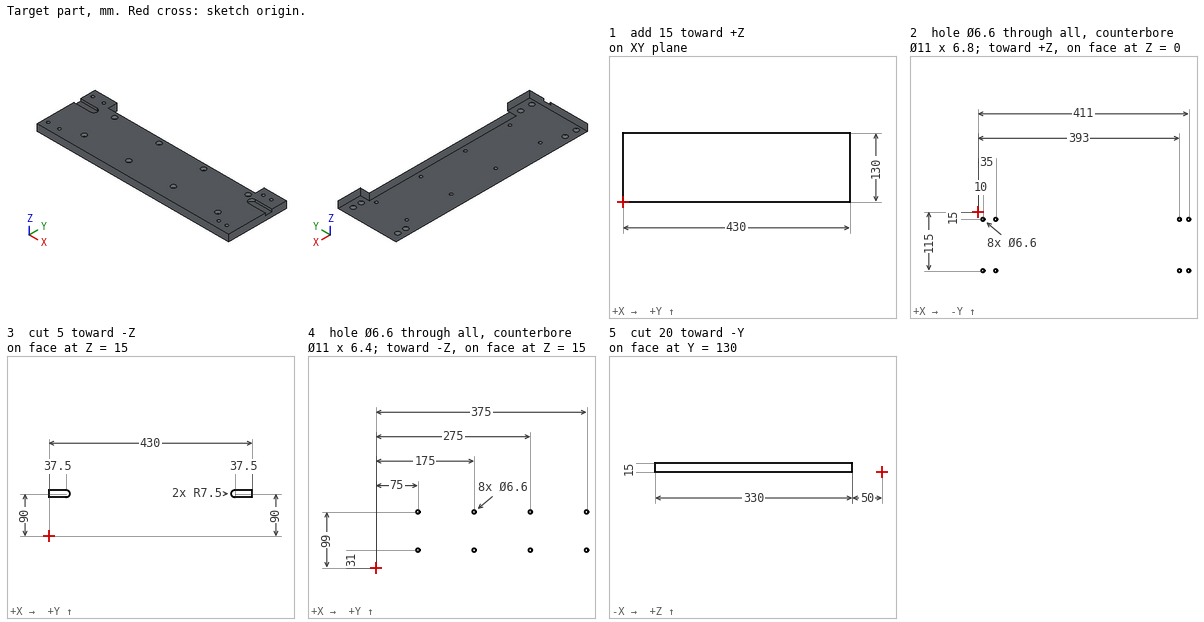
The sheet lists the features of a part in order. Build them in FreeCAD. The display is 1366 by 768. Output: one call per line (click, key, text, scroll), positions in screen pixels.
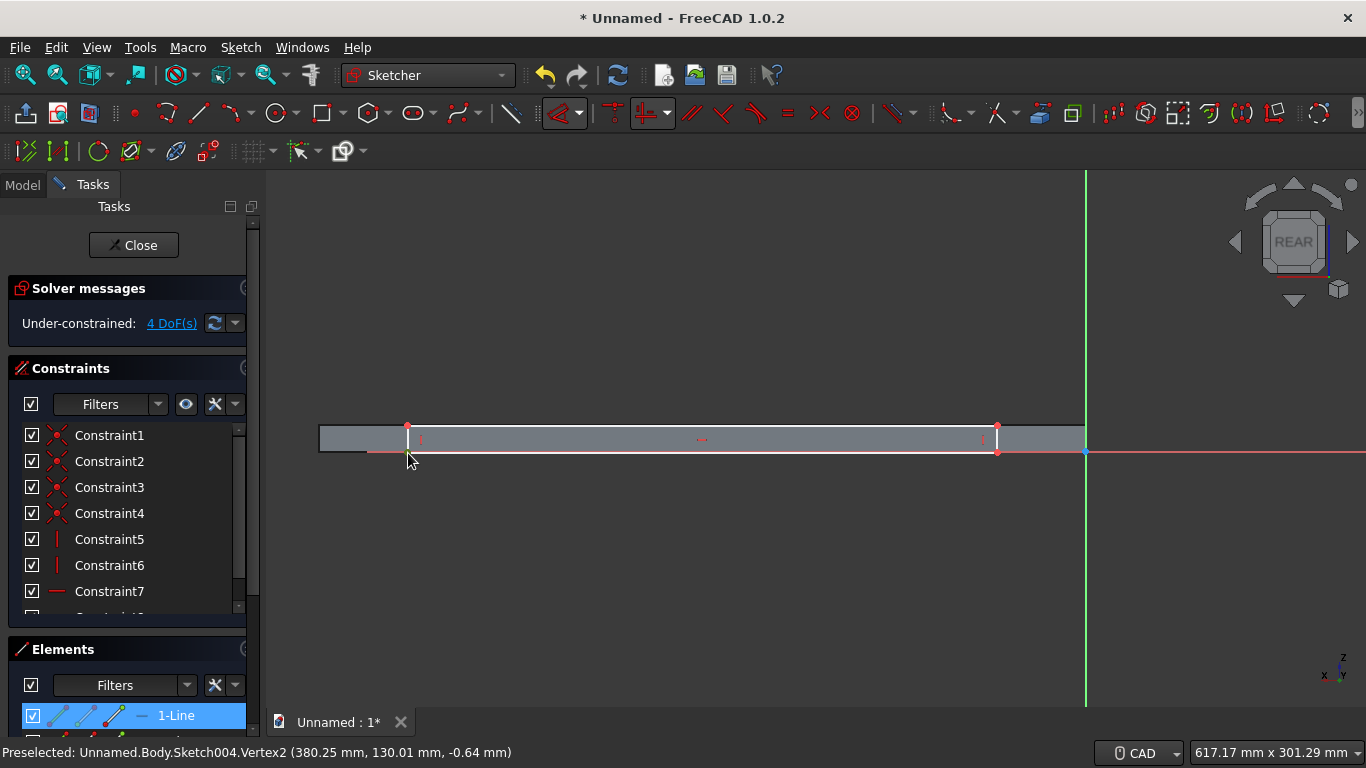
click(1136, 452)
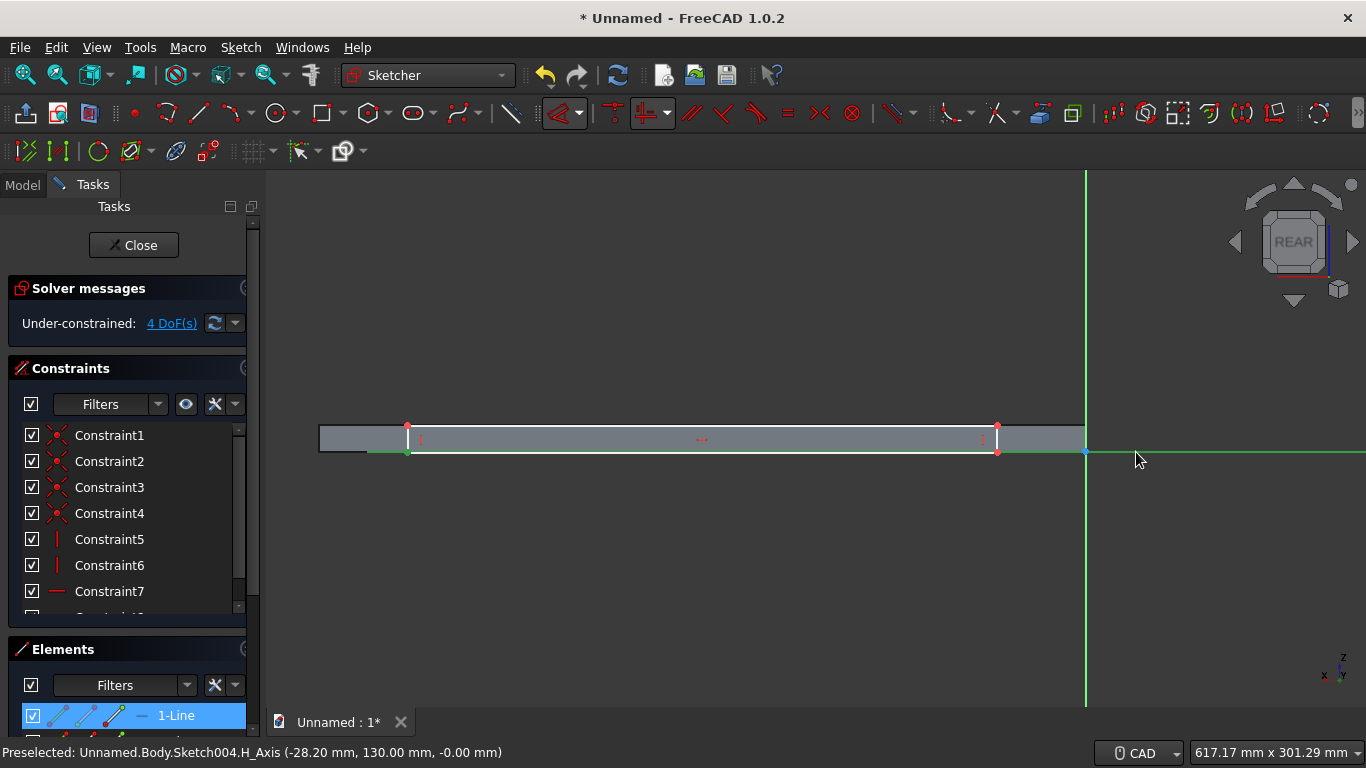
click(614, 114)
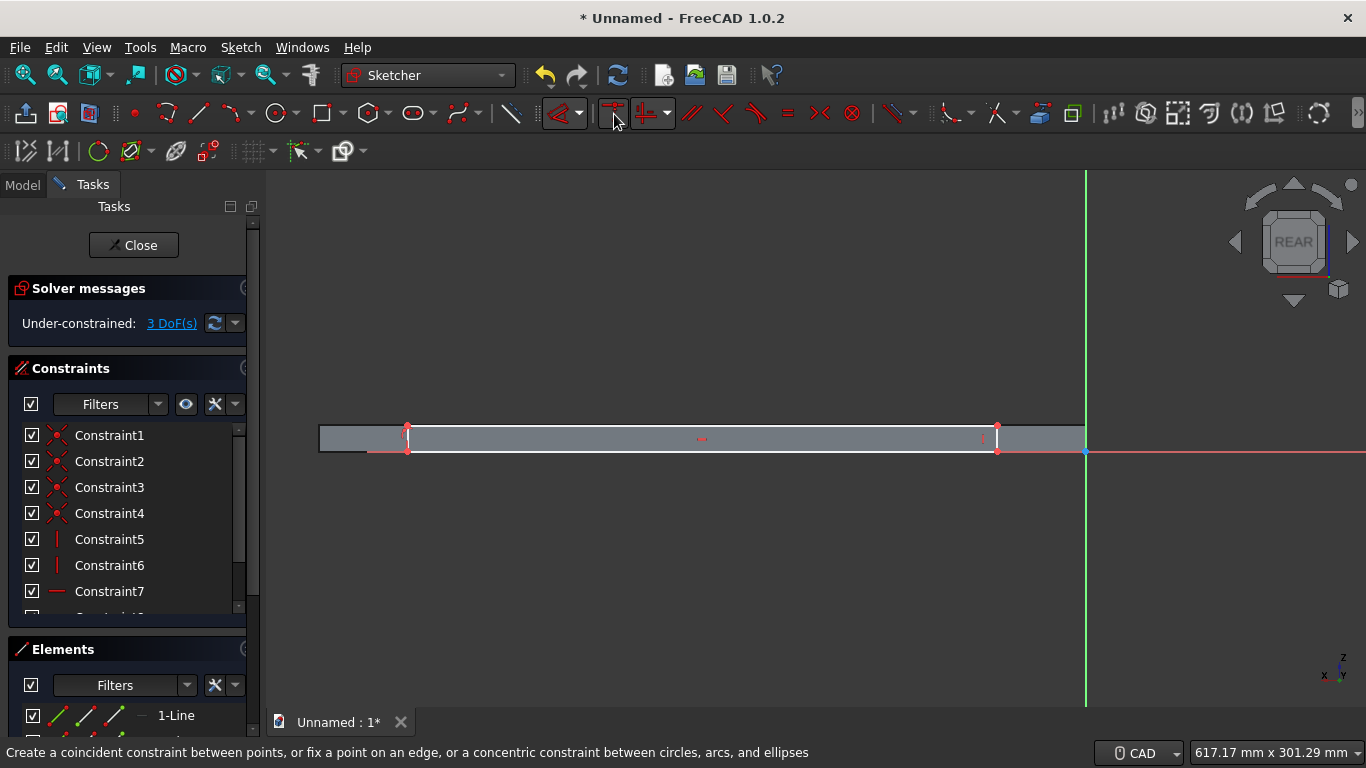
scroll(408, 436, up, 2)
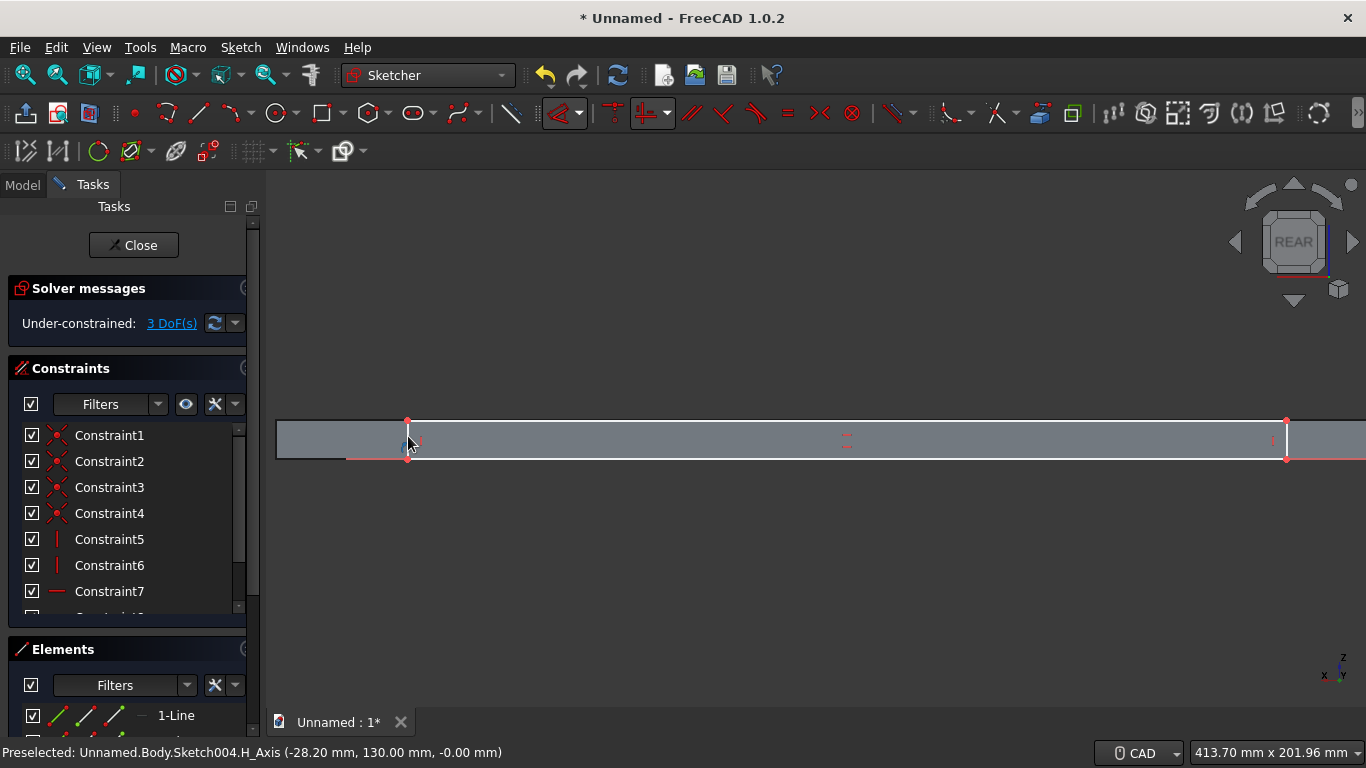
click(408, 436)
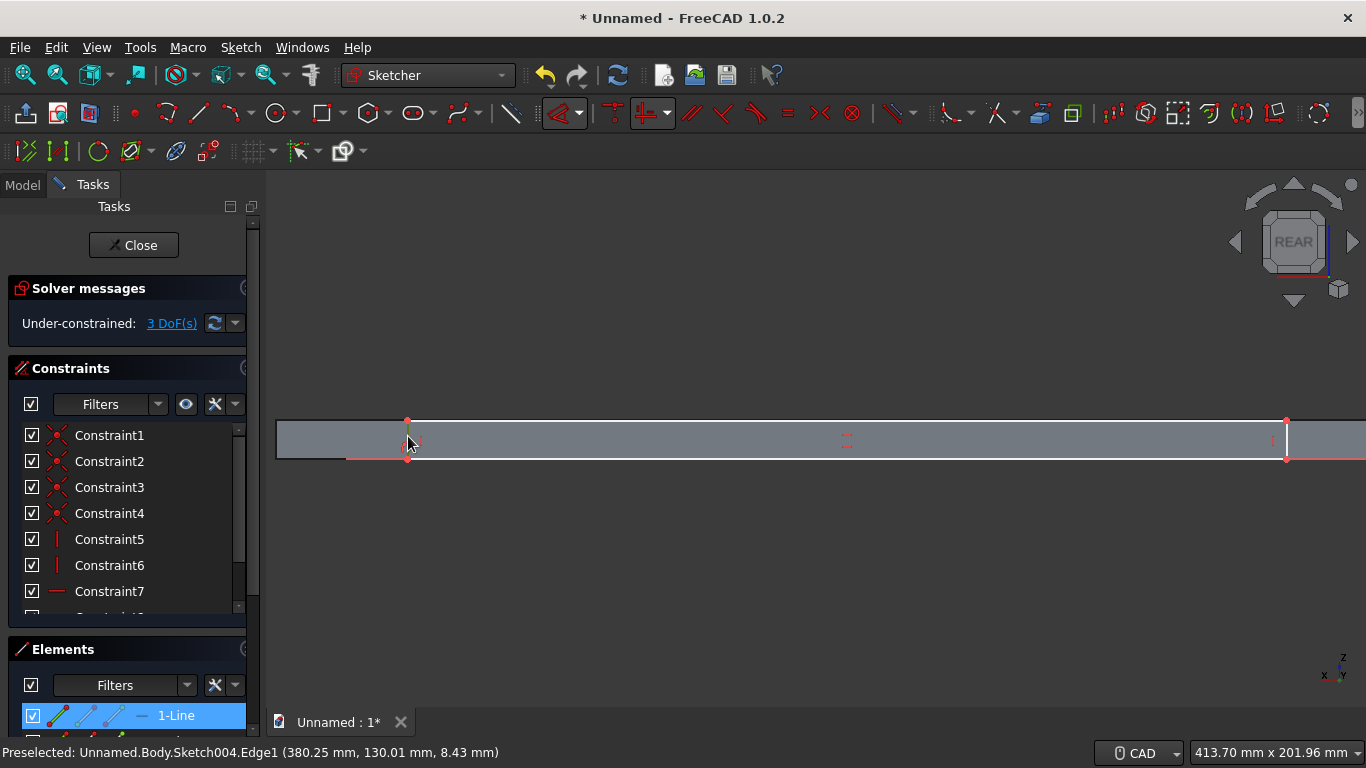
key(i)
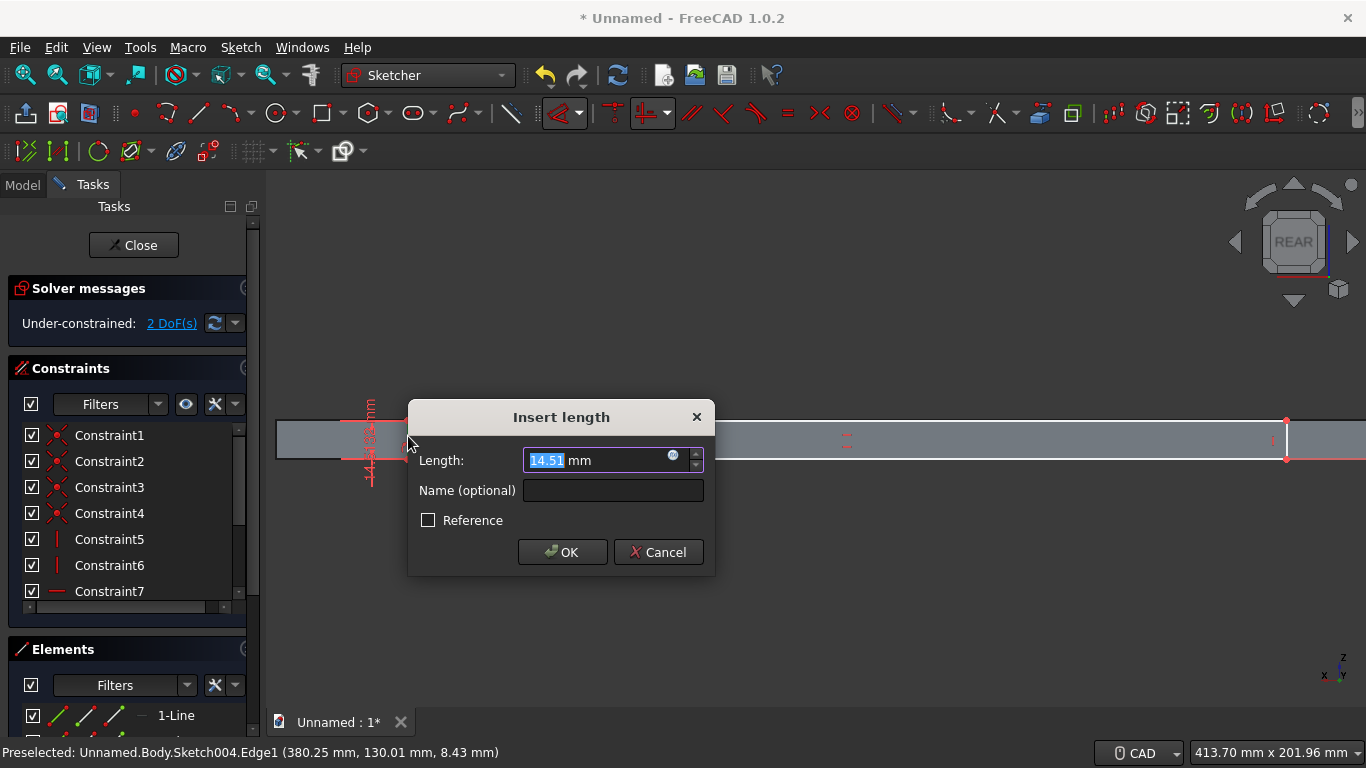
text(15)
key(Return)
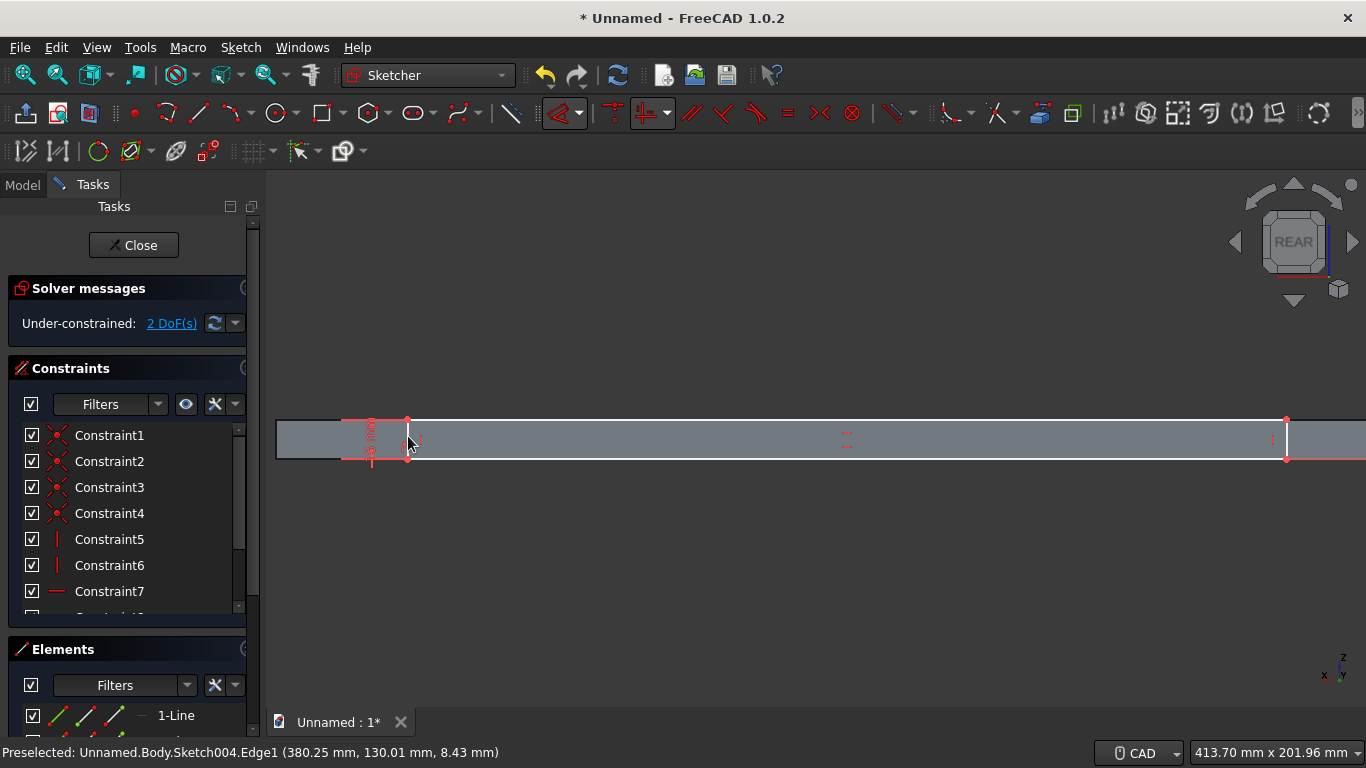
click(672, 459)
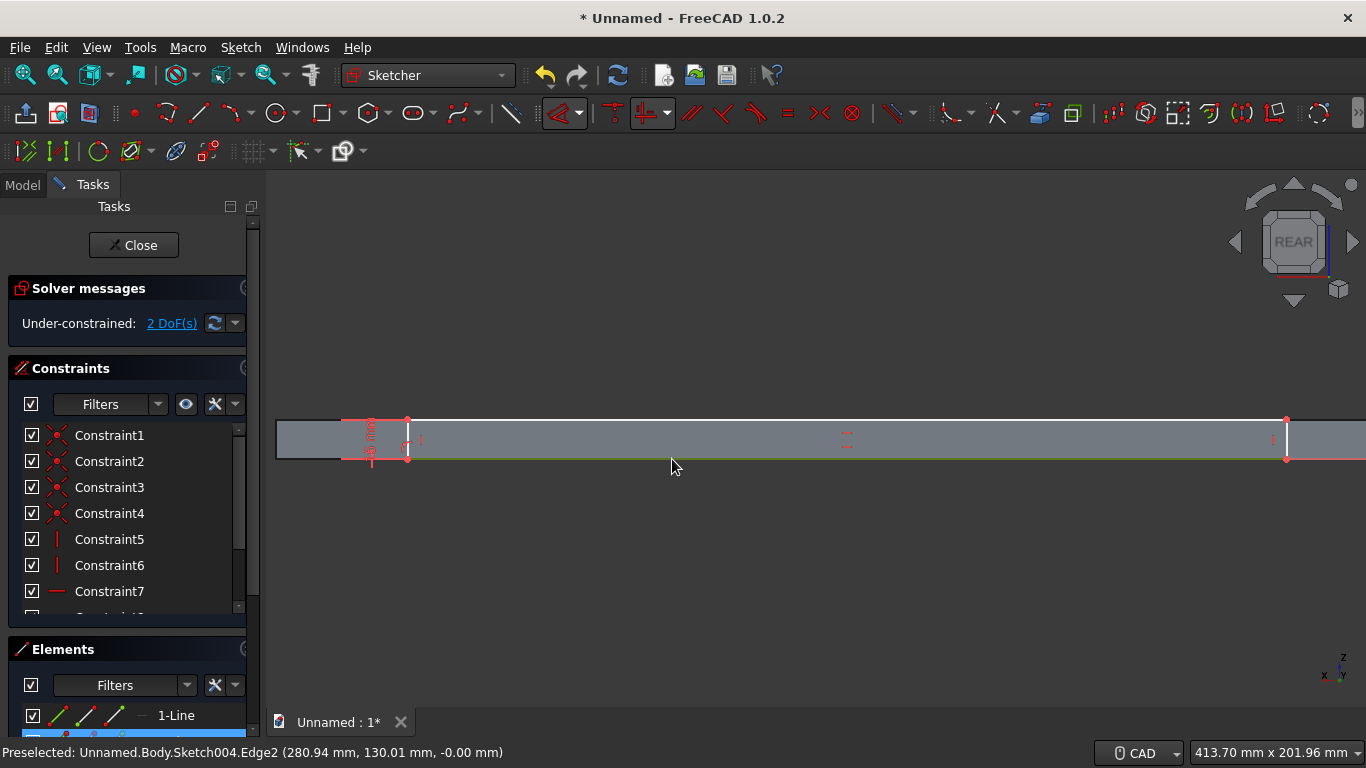
click(582, 114)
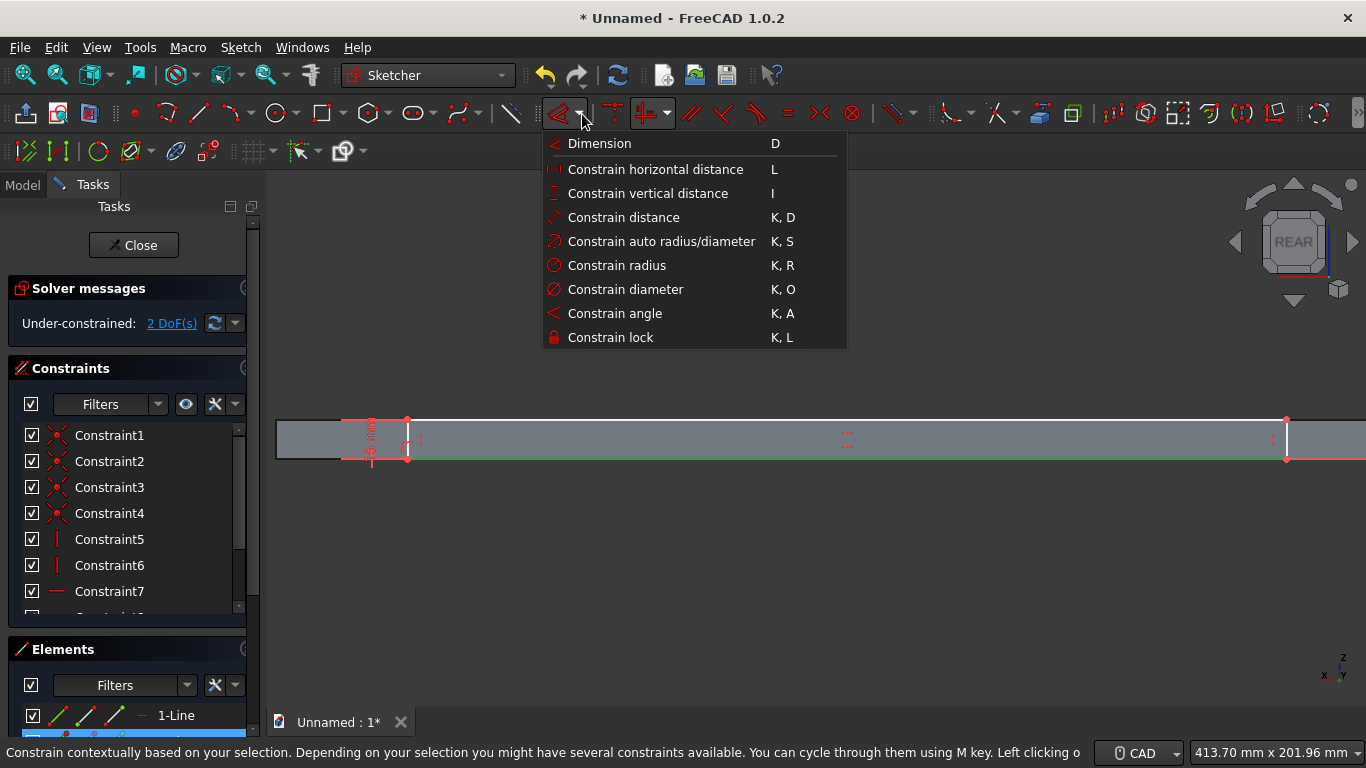
click(695, 169)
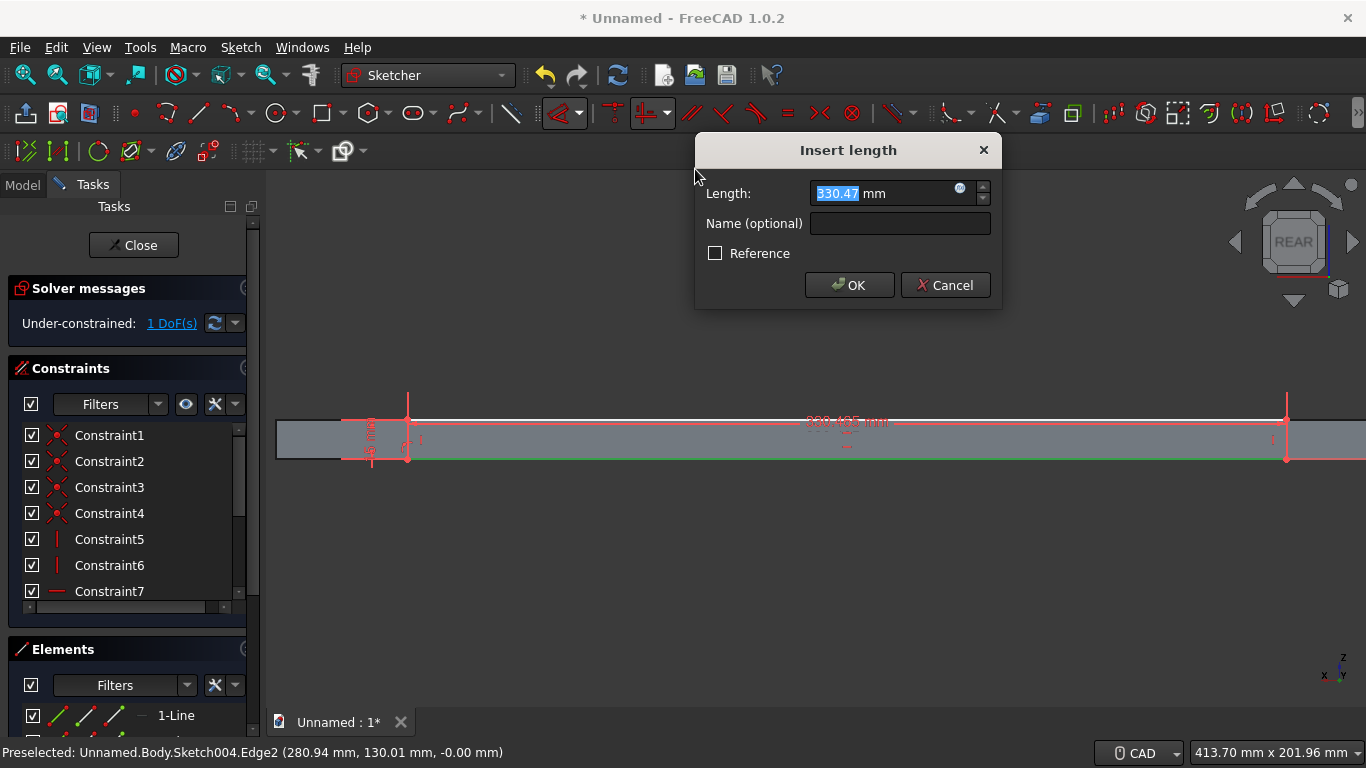
text(330)
key(Return)